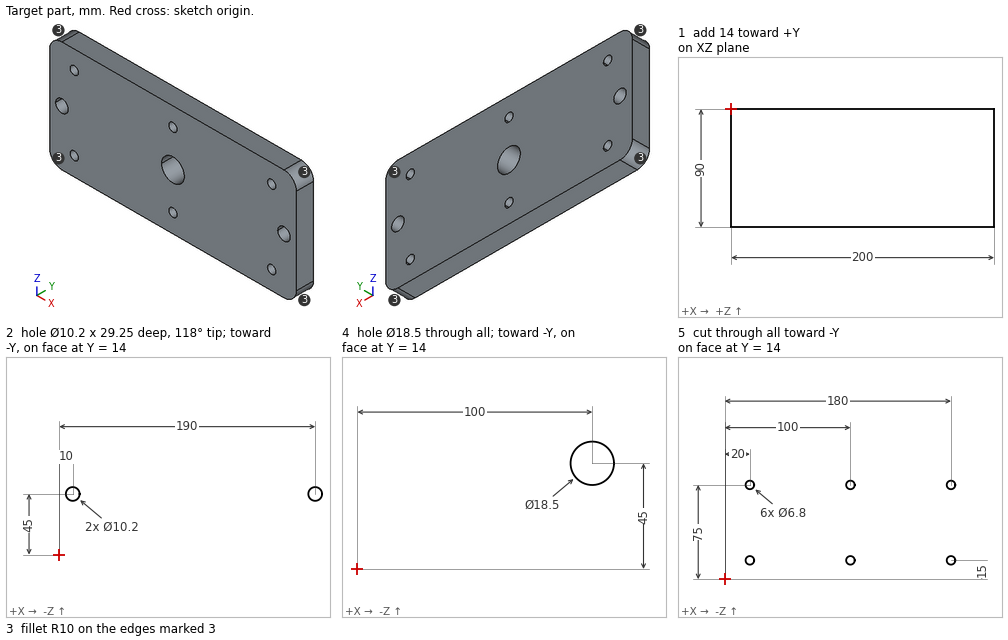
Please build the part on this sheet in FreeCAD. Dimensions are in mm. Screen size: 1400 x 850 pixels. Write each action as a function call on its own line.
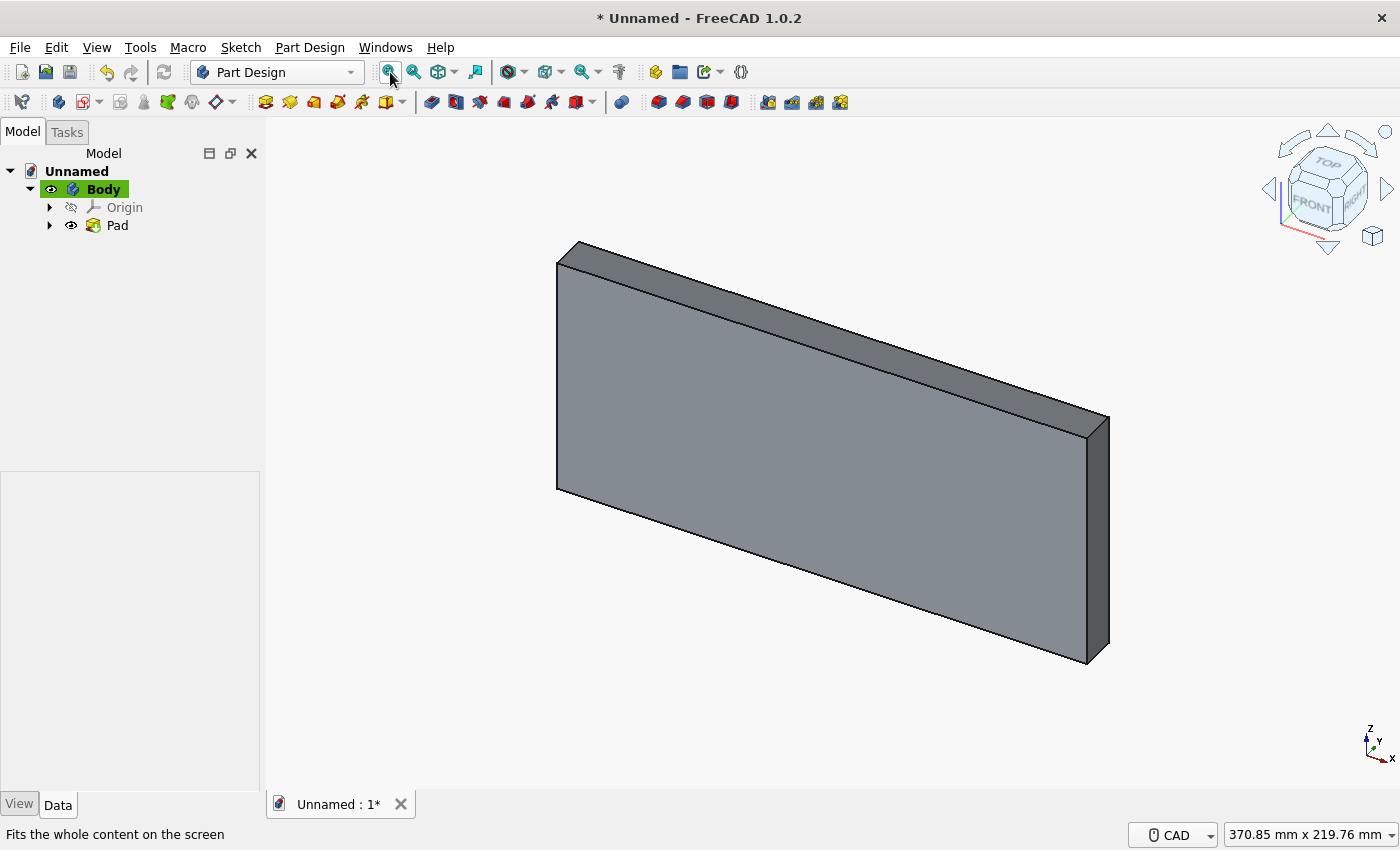
key(4)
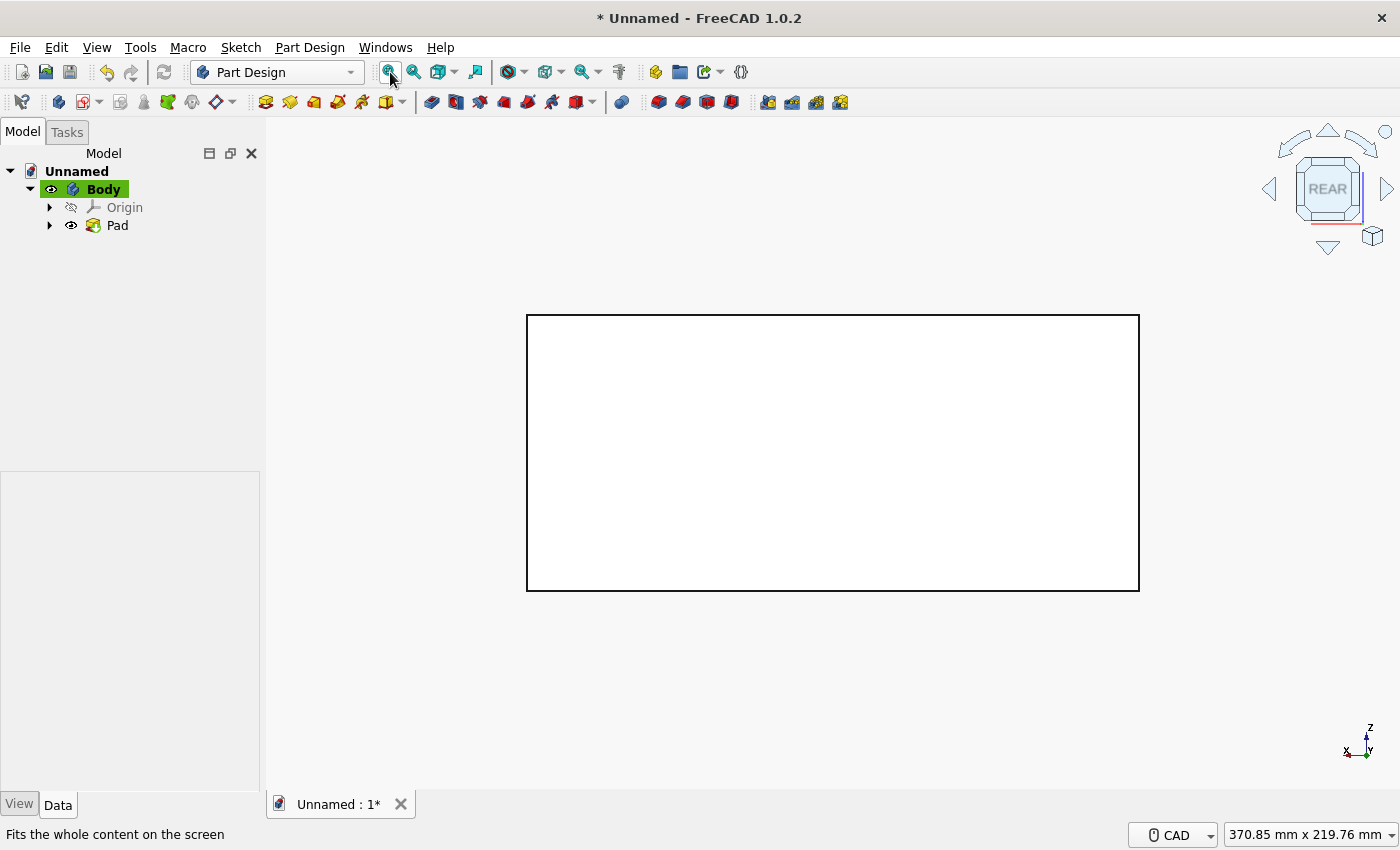
click(746, 452)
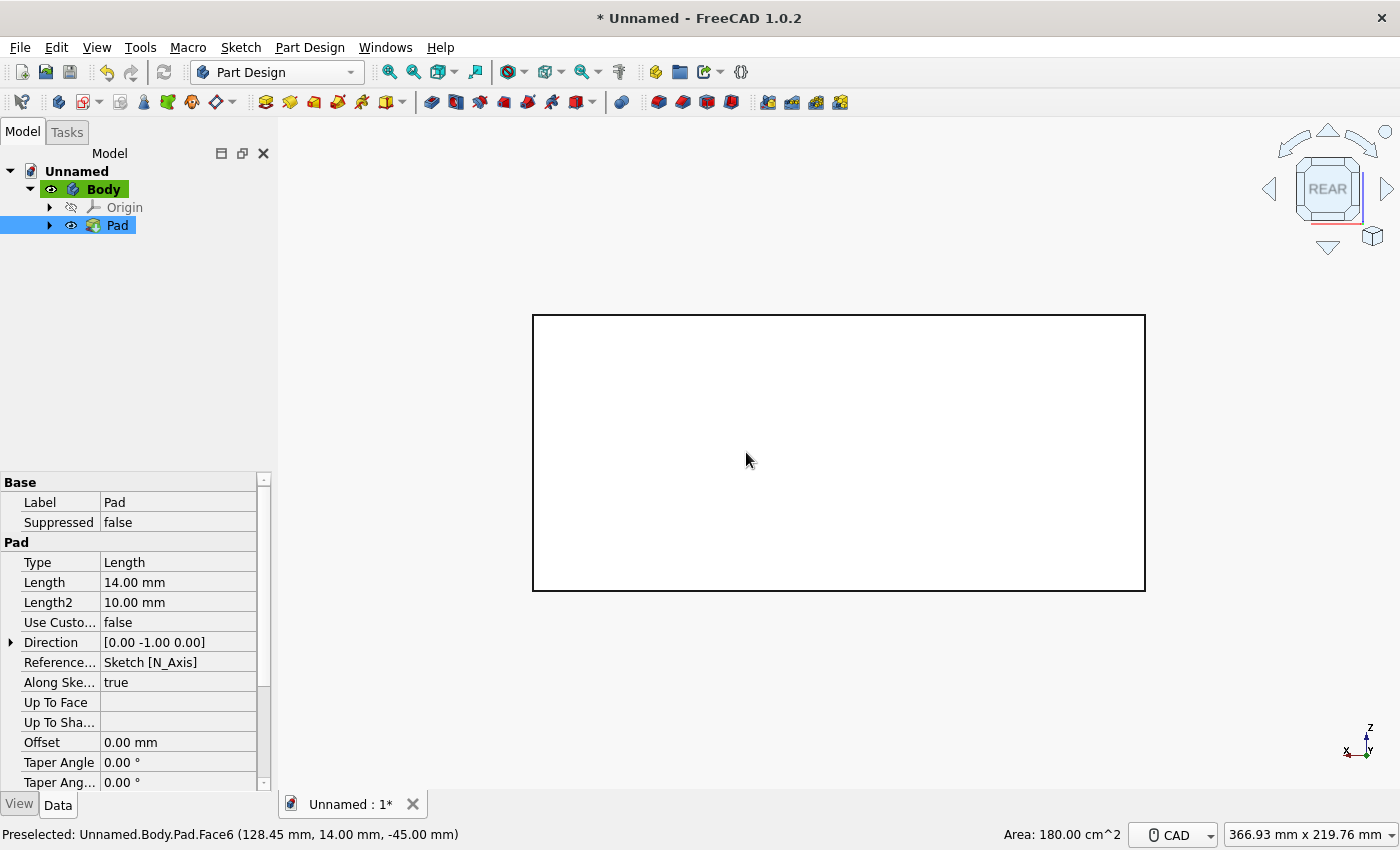
click(84, 102)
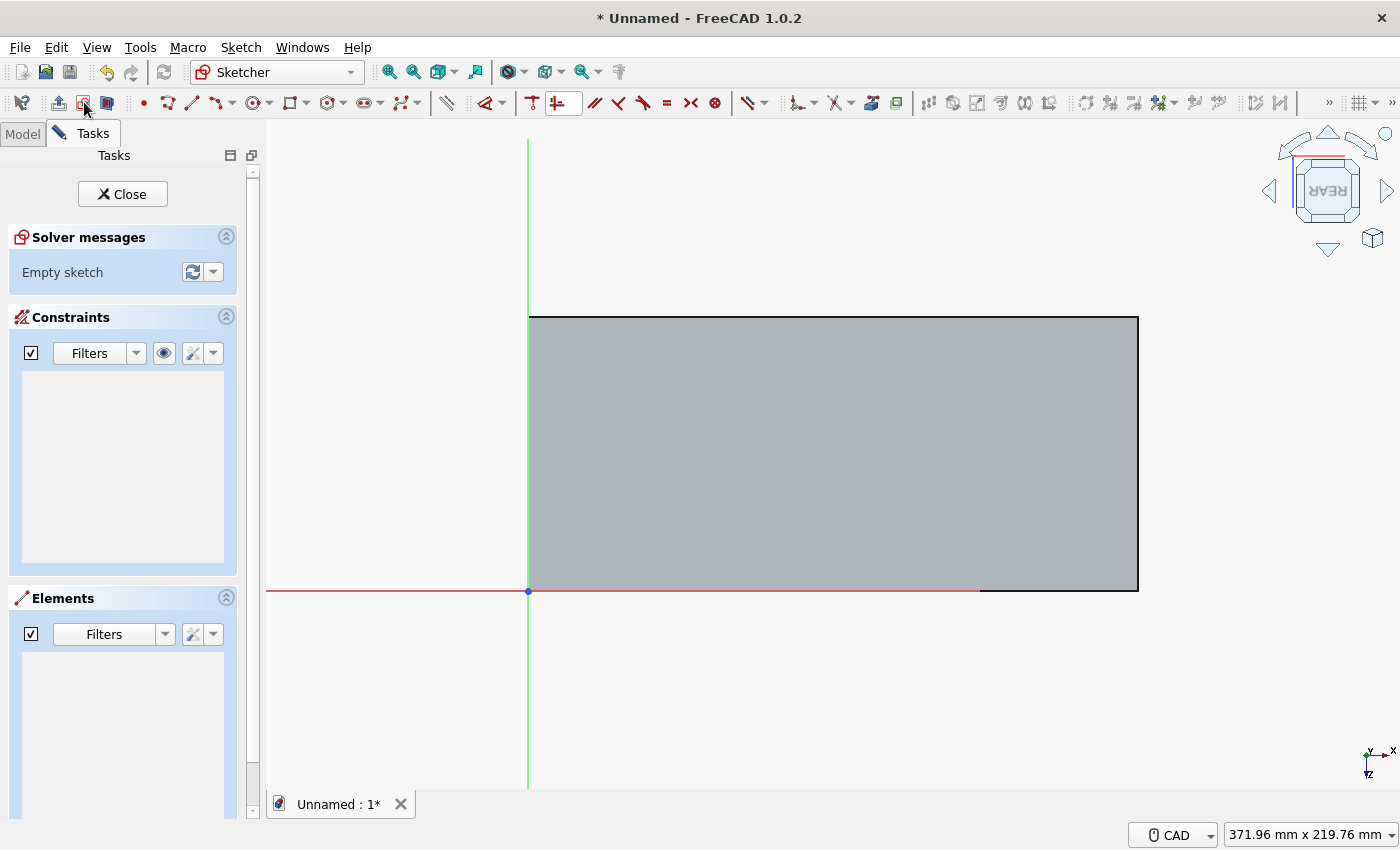
click(254, 104)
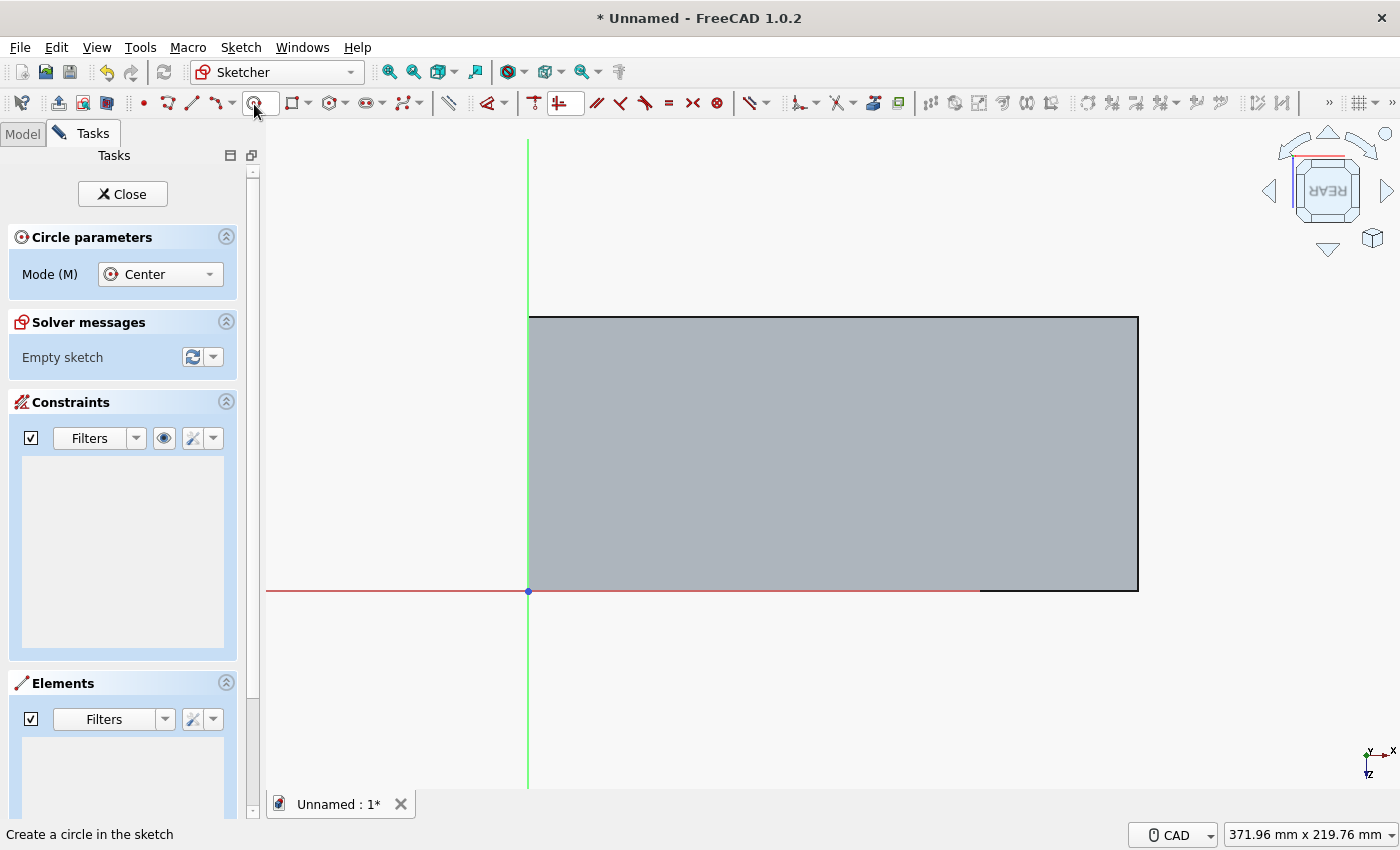
scroll(559, 454, up, 2)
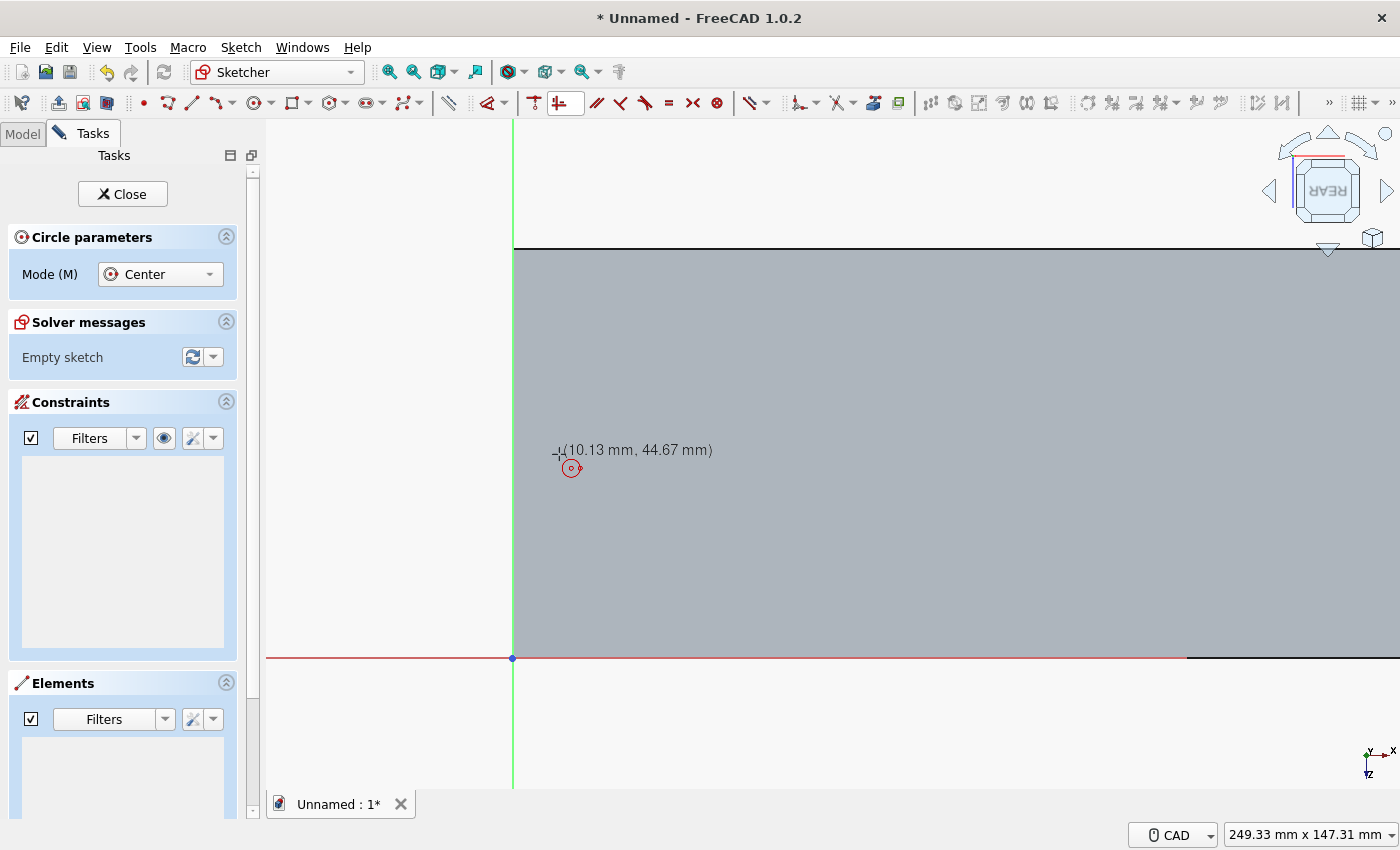
click(558, 454)
click(575, 437)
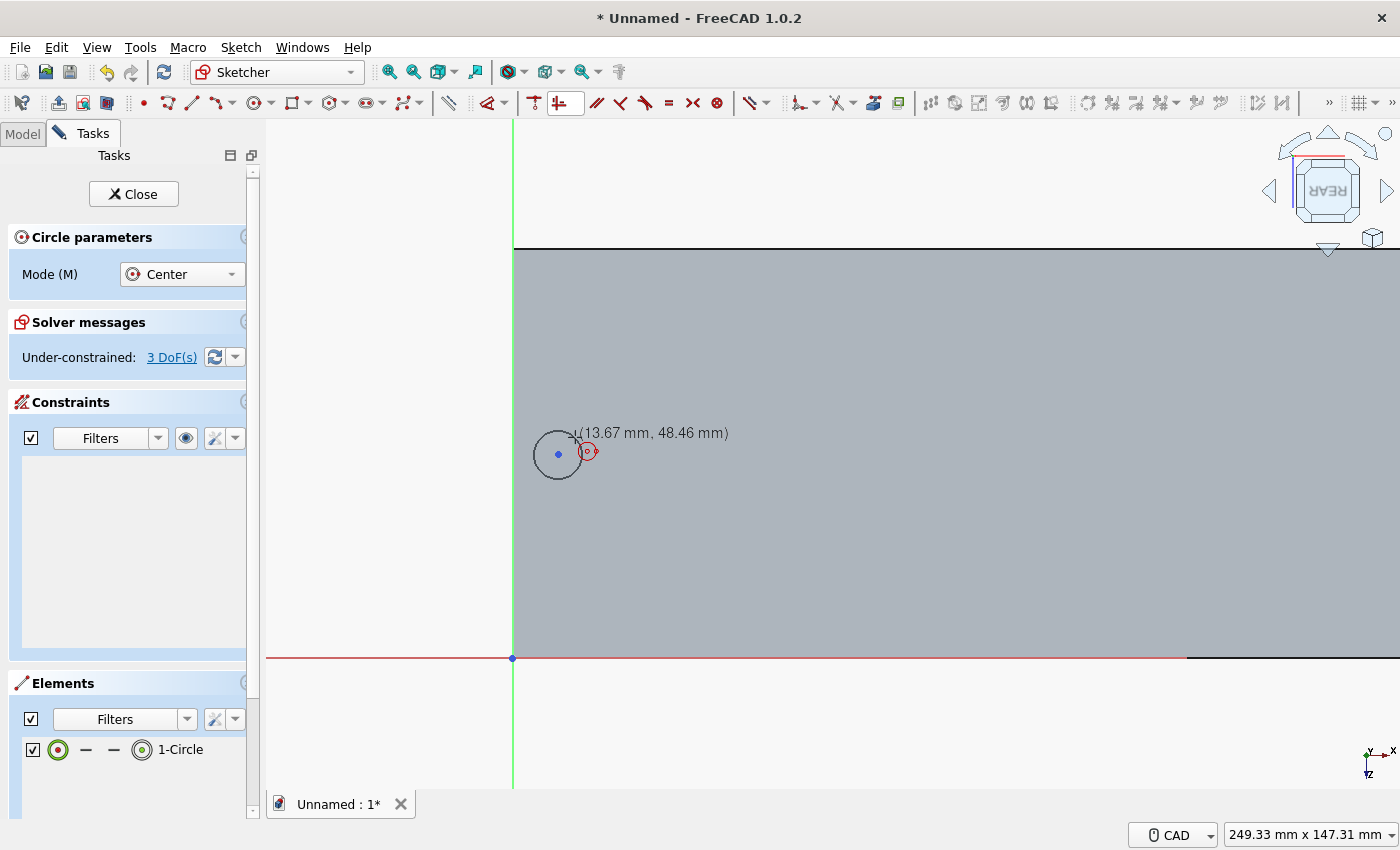
scroll(294, 147, down, 1)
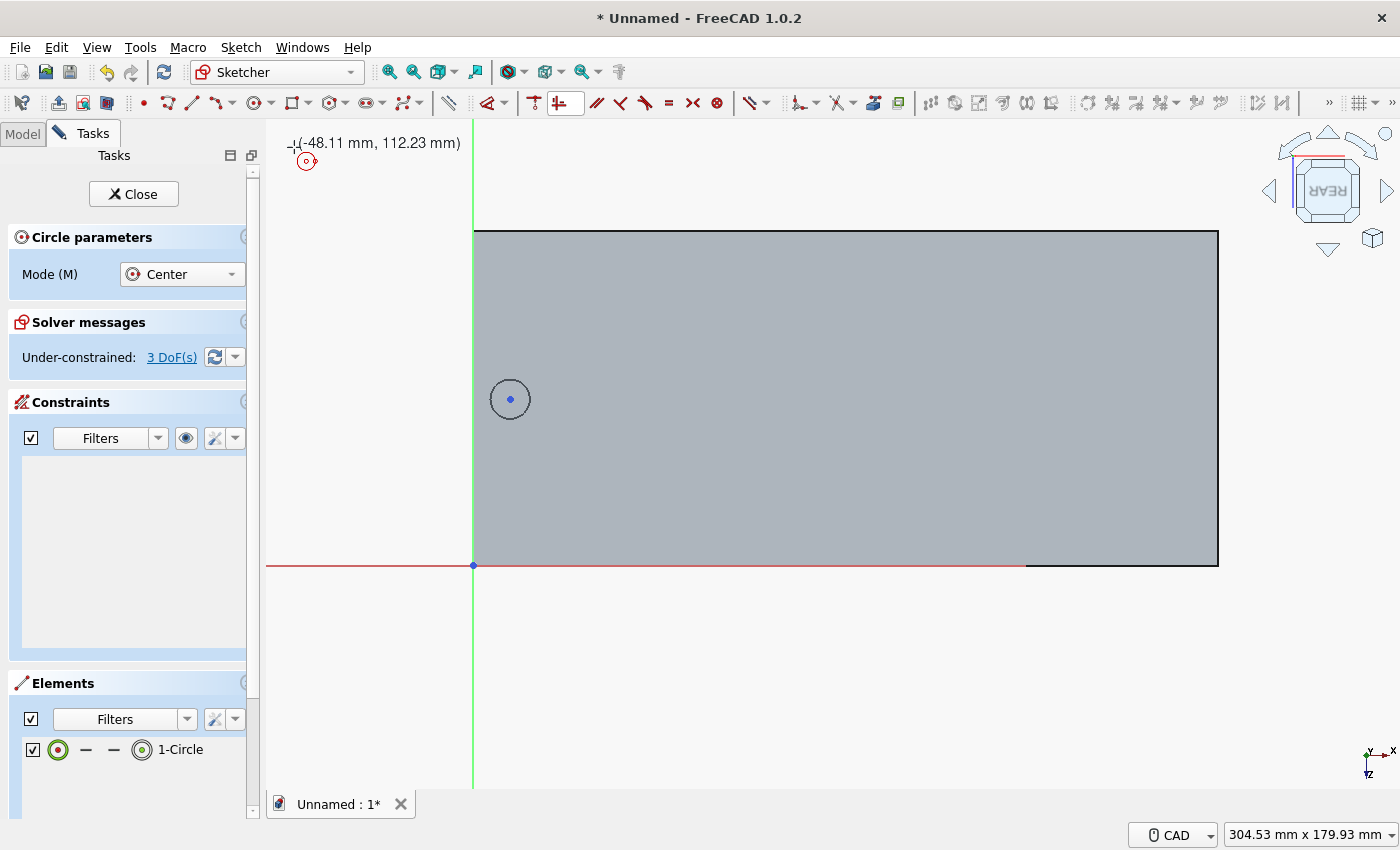
click(1181, 398)
click(1194, 385)
key(Escape)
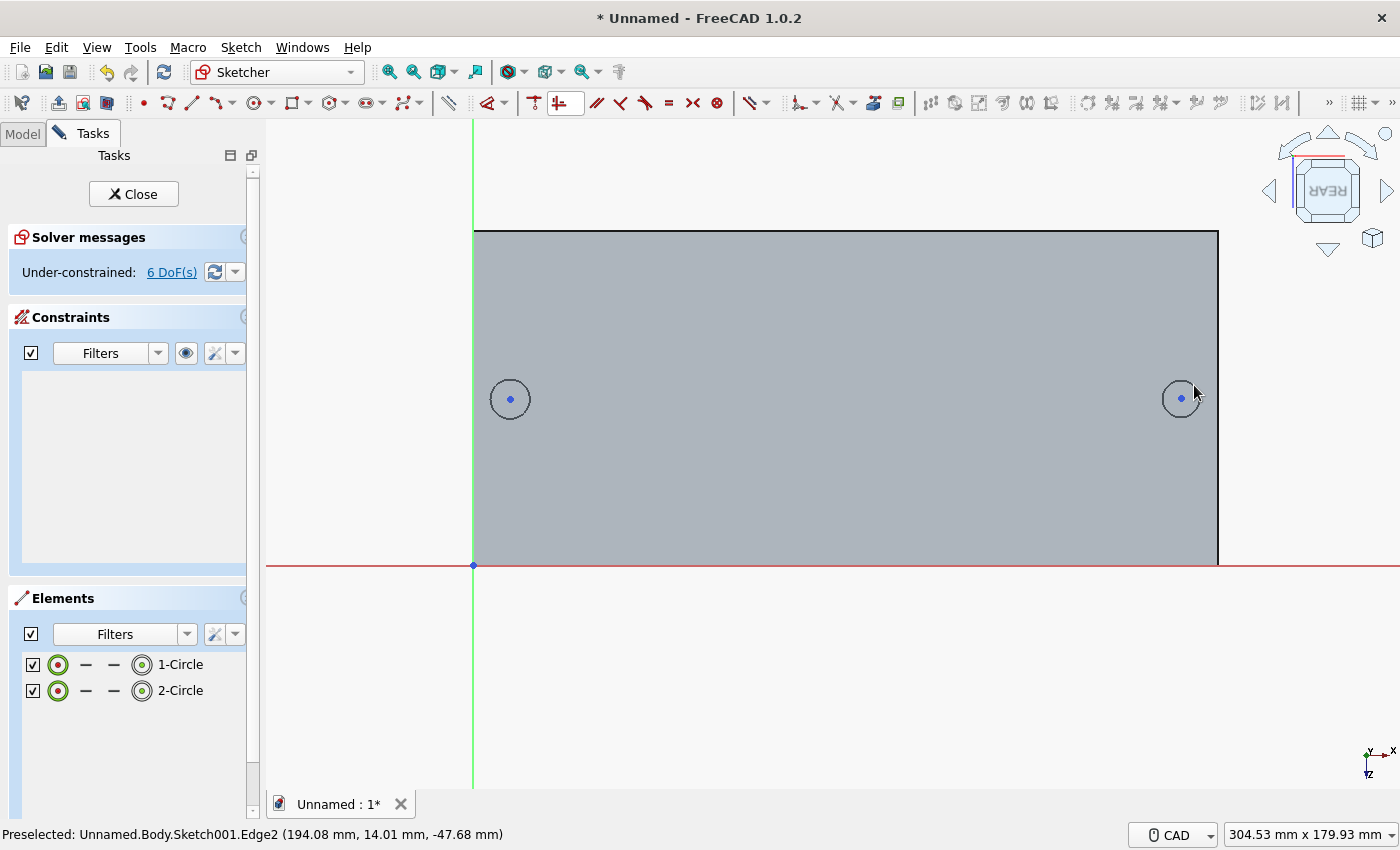
click(524, 385)